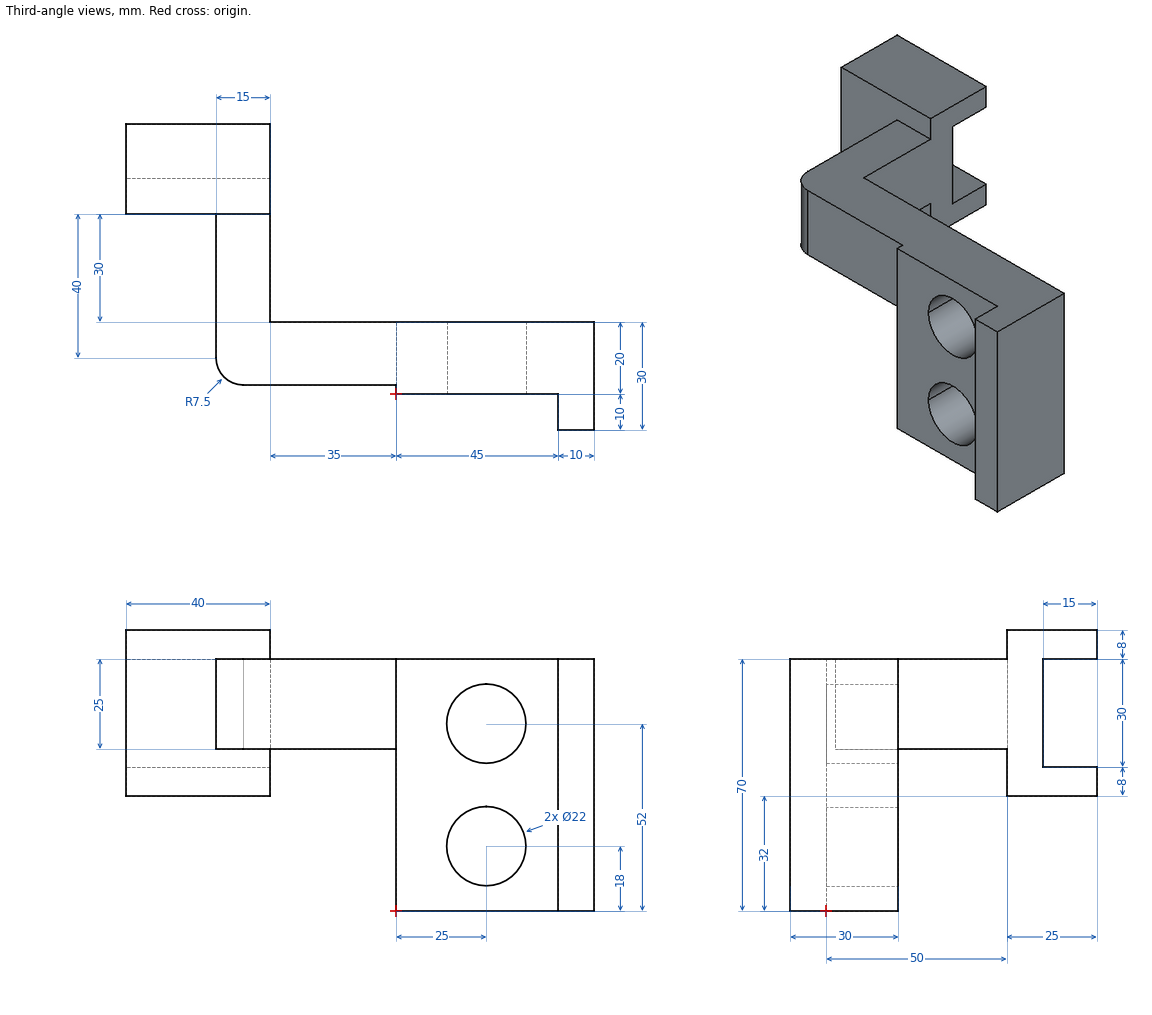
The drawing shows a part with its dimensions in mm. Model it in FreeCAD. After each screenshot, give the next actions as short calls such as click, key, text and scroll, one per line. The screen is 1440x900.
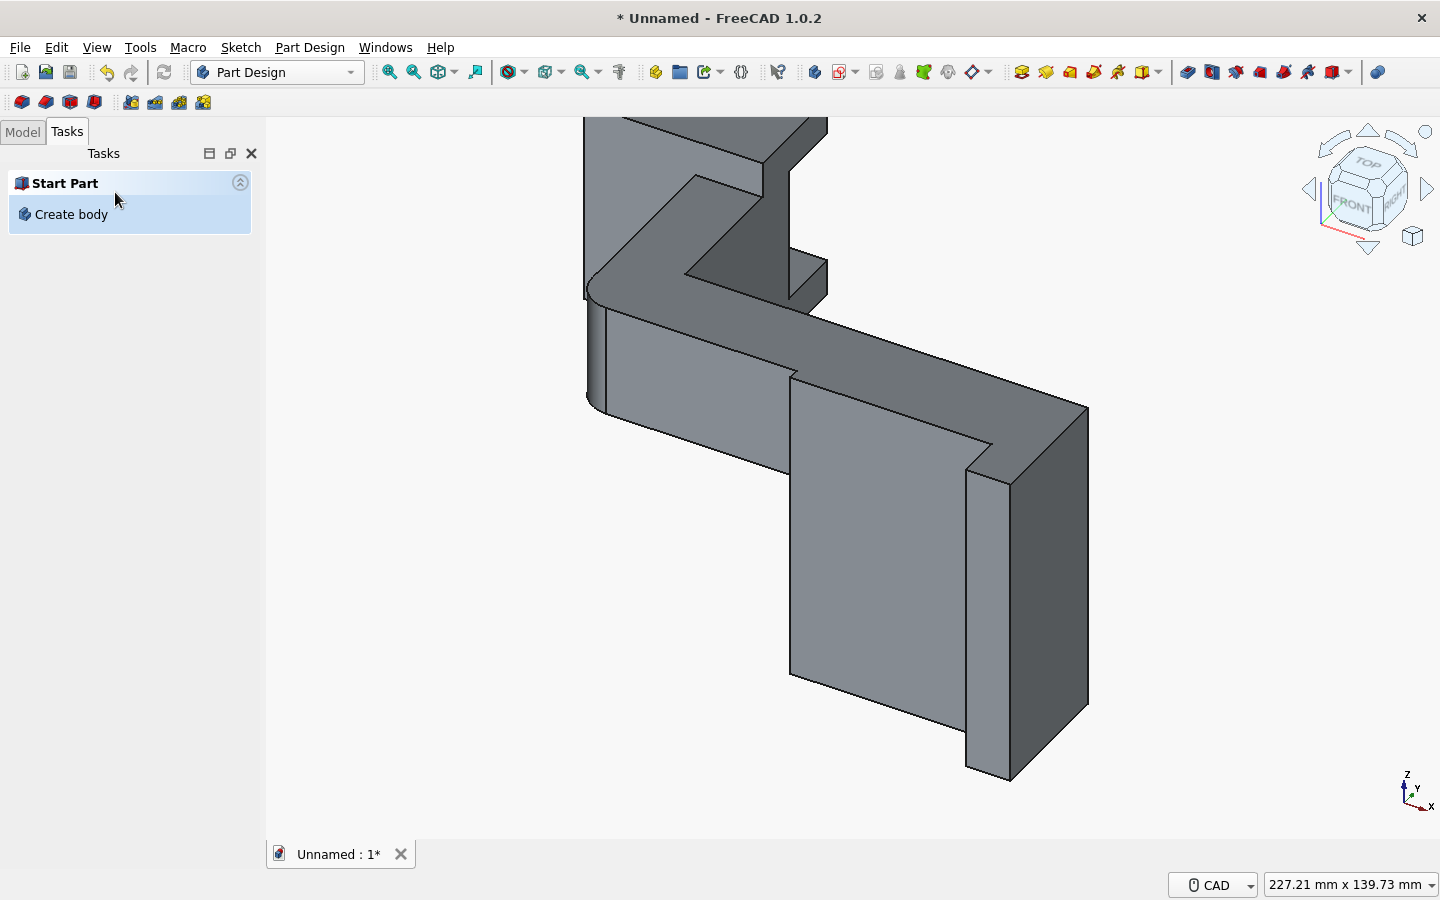
click(390, 72)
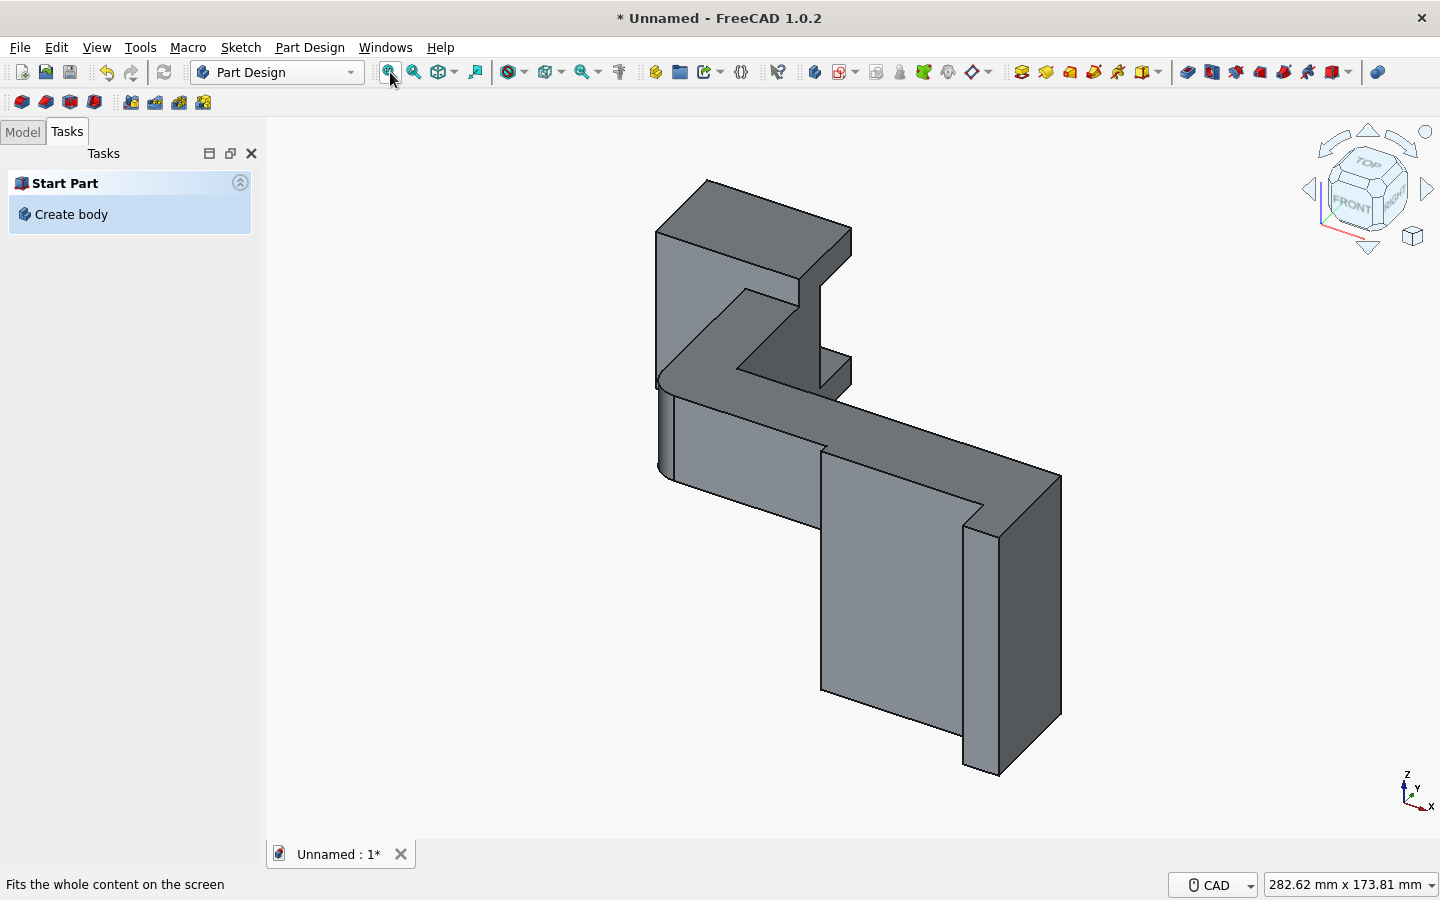
key(4)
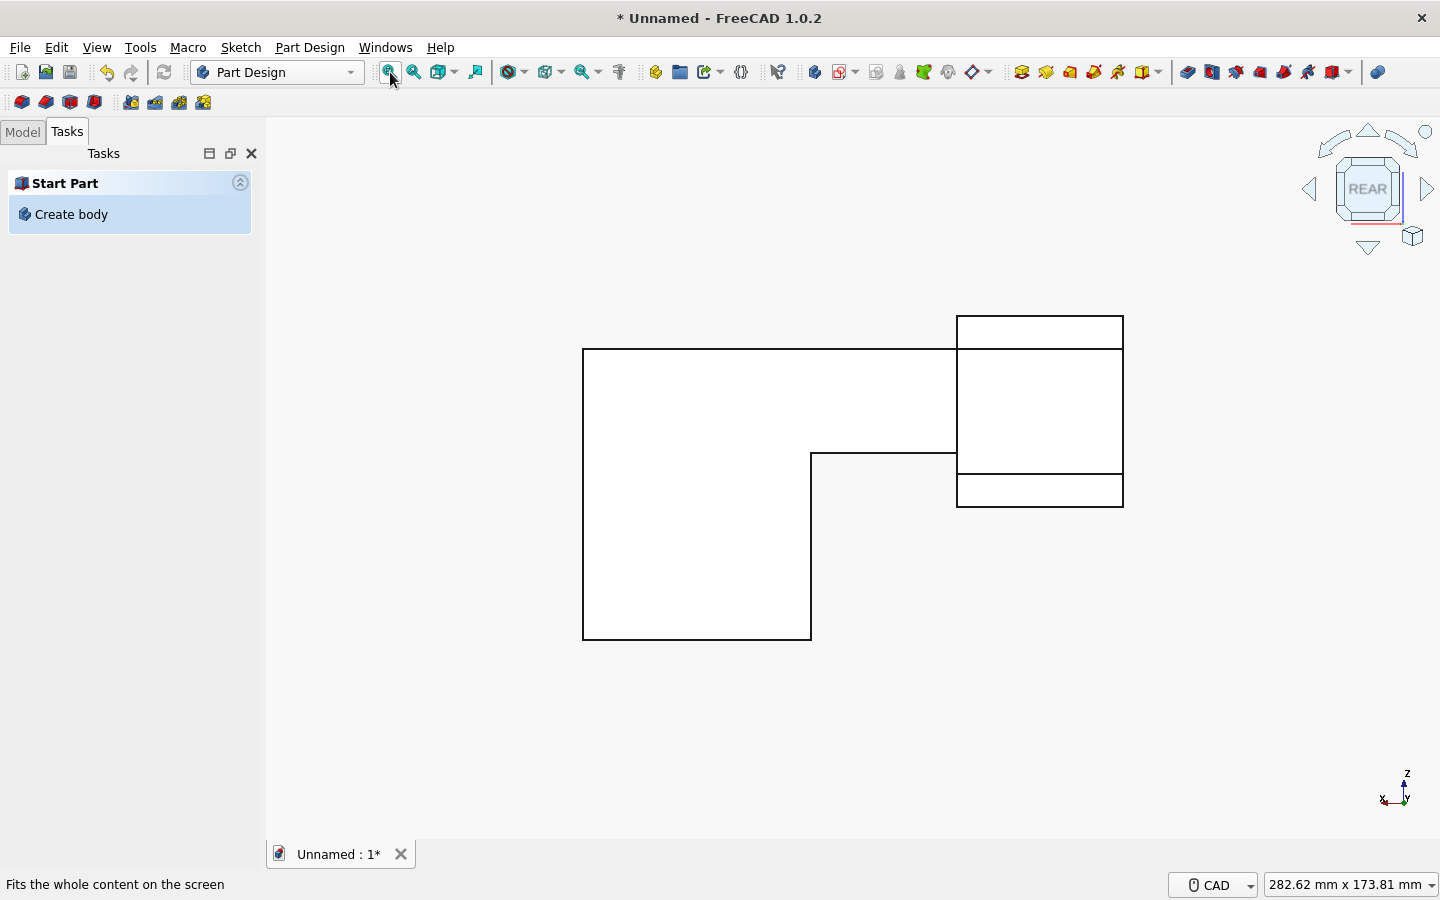
click(717, 452)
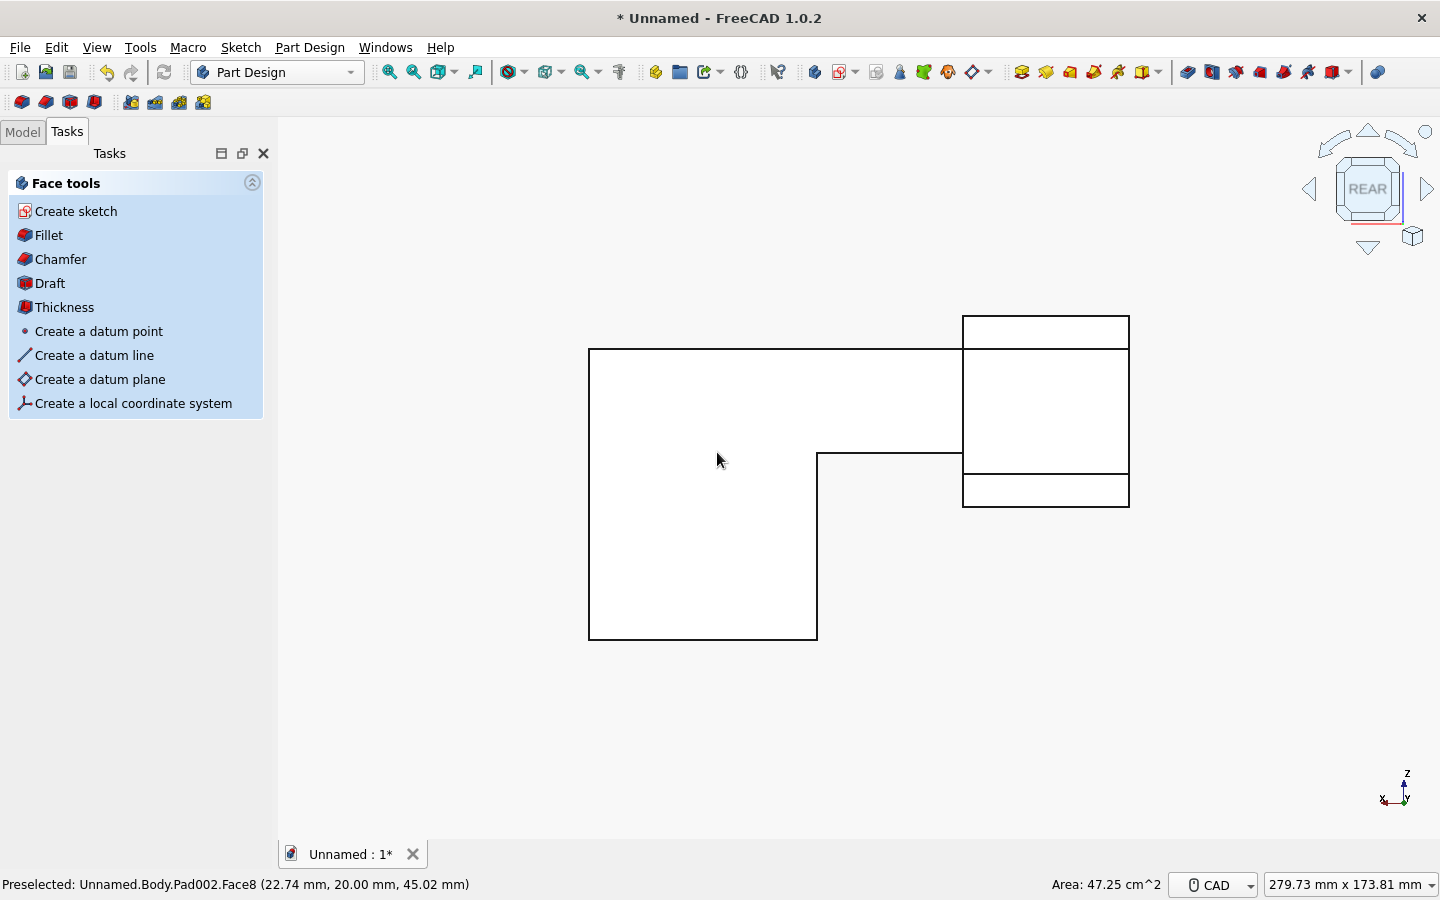
click(840, 72)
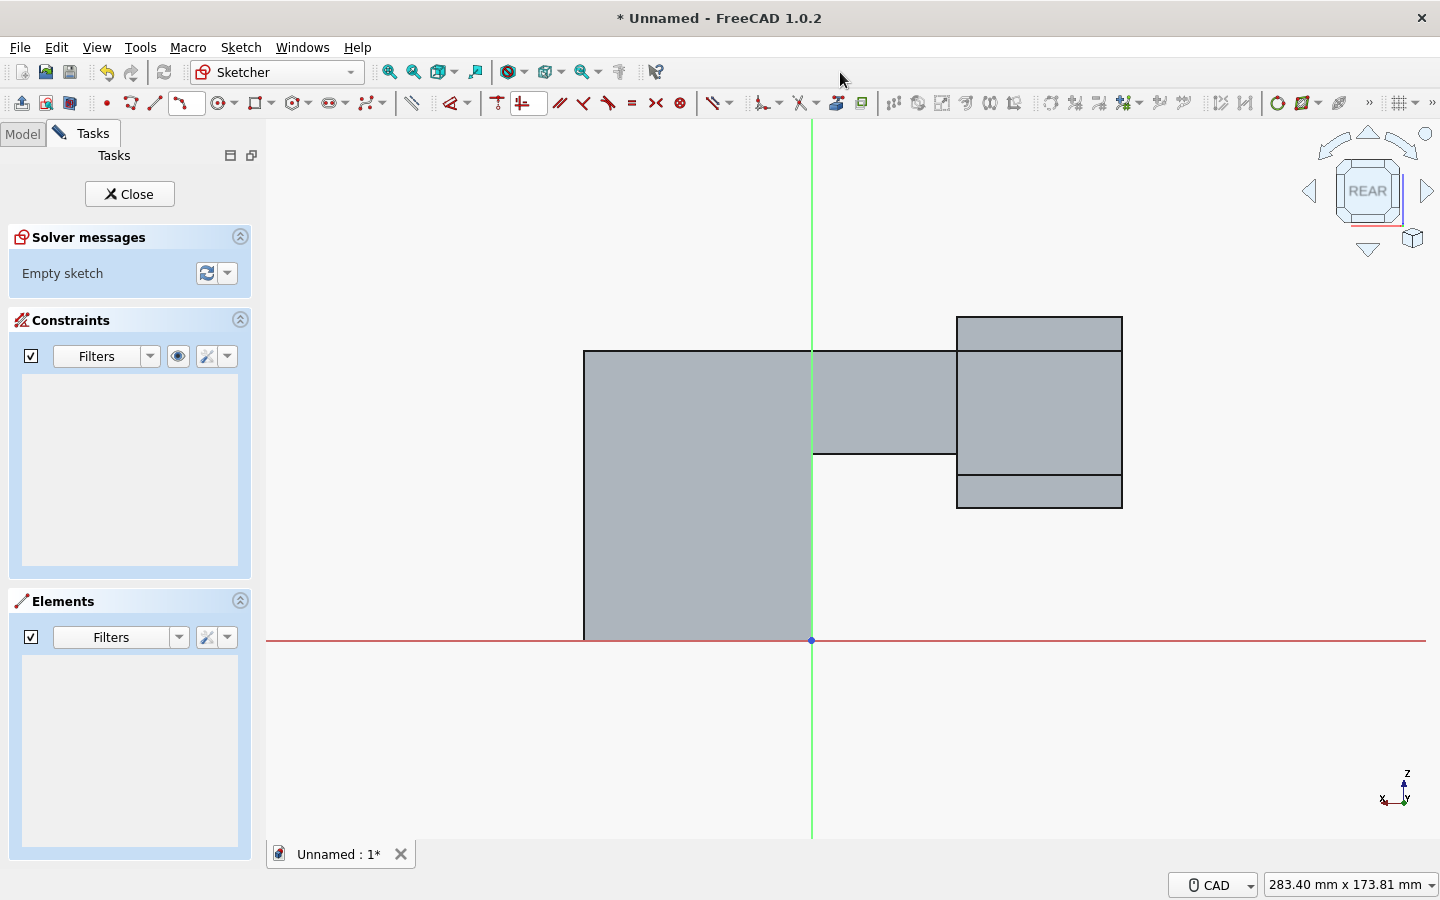
scroll(679, 548, up, 3)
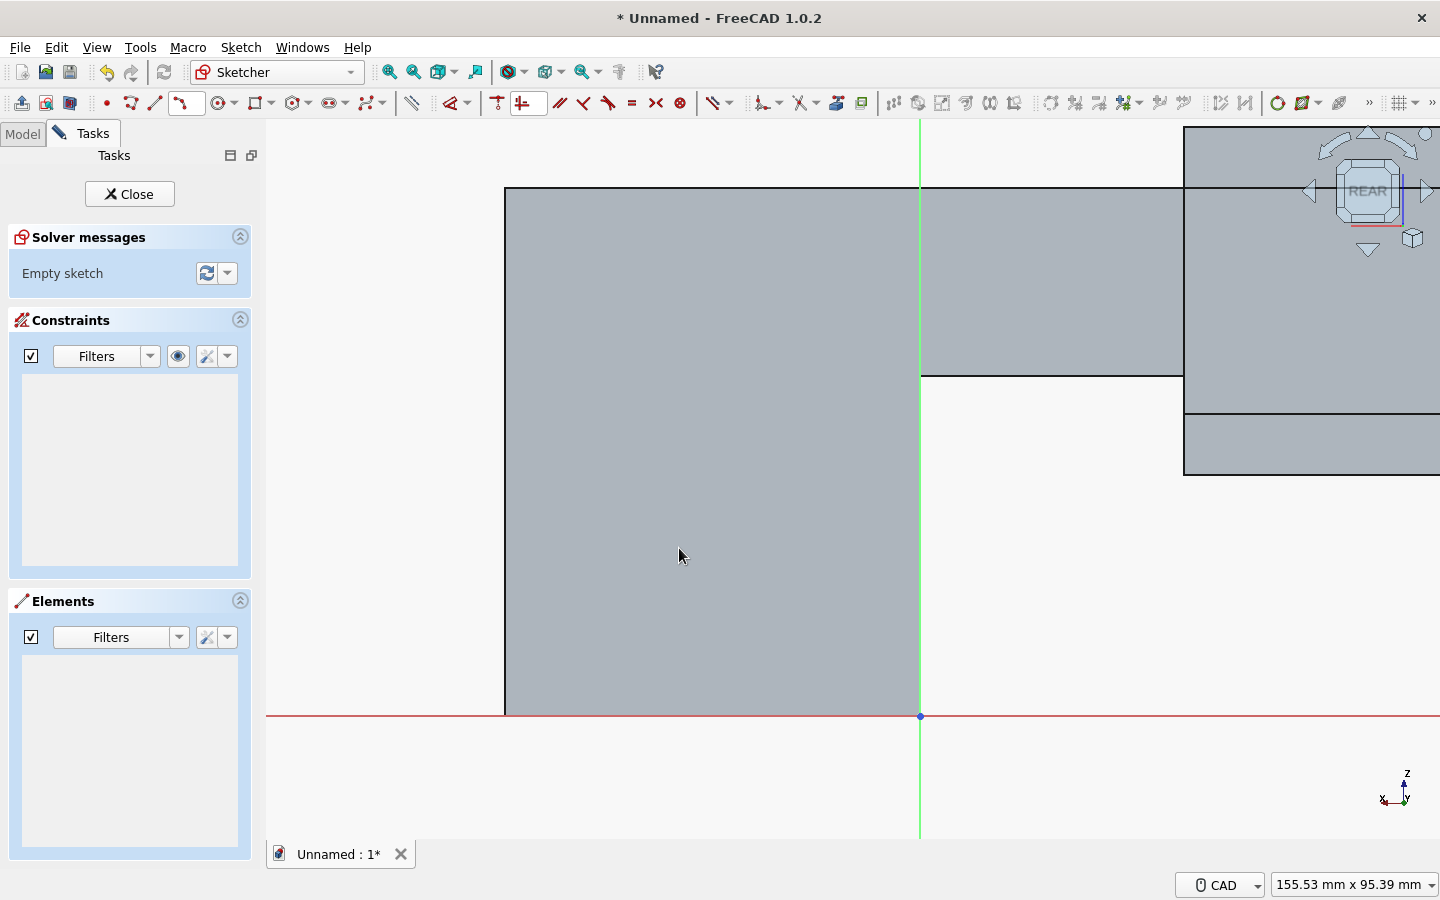
click(218, 104)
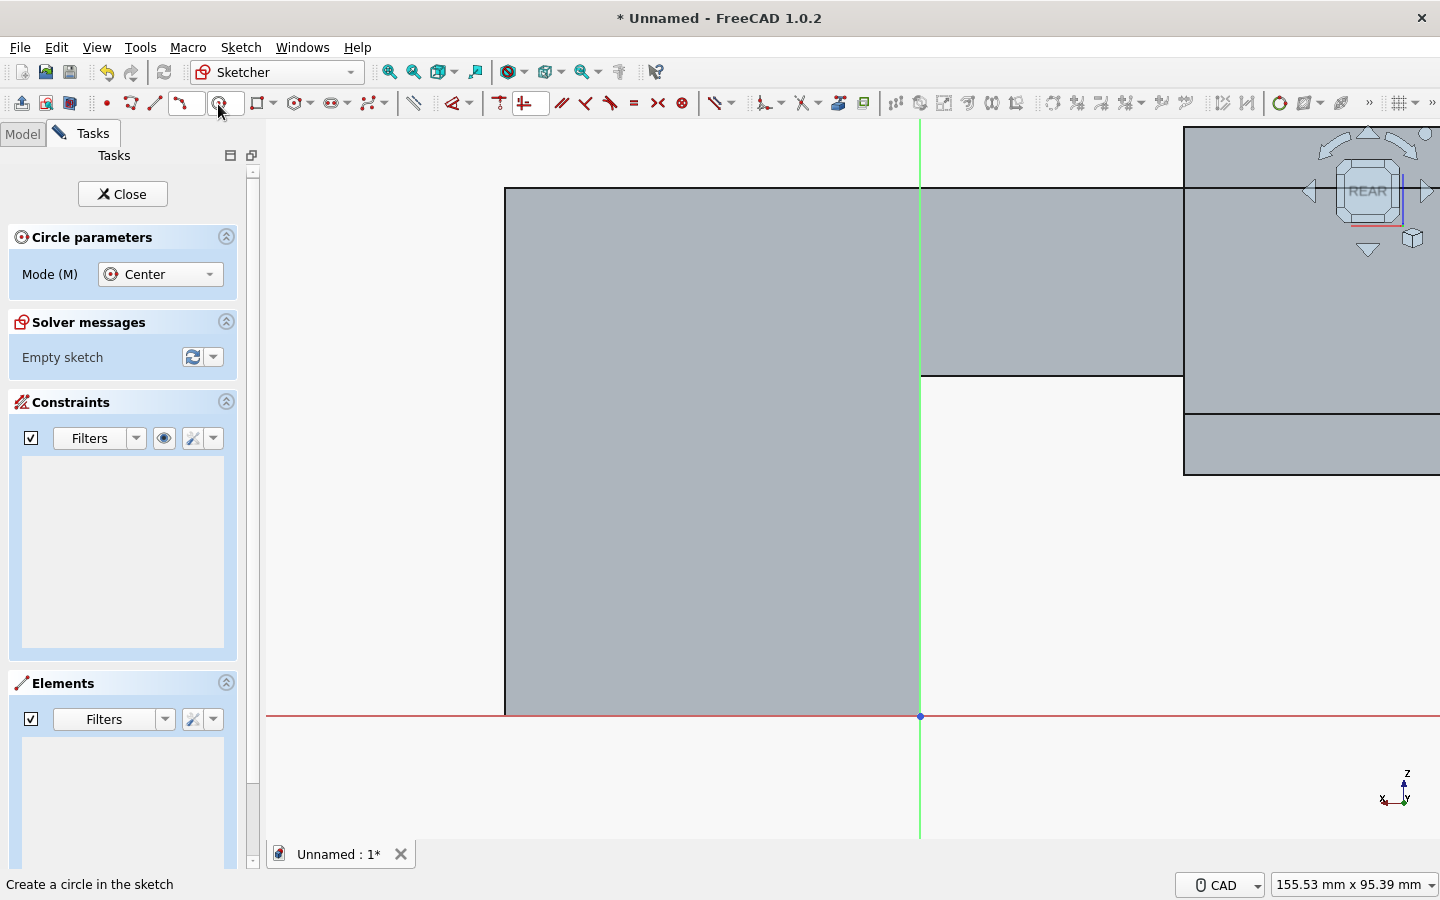
click(732, 580)
click(790, 522)